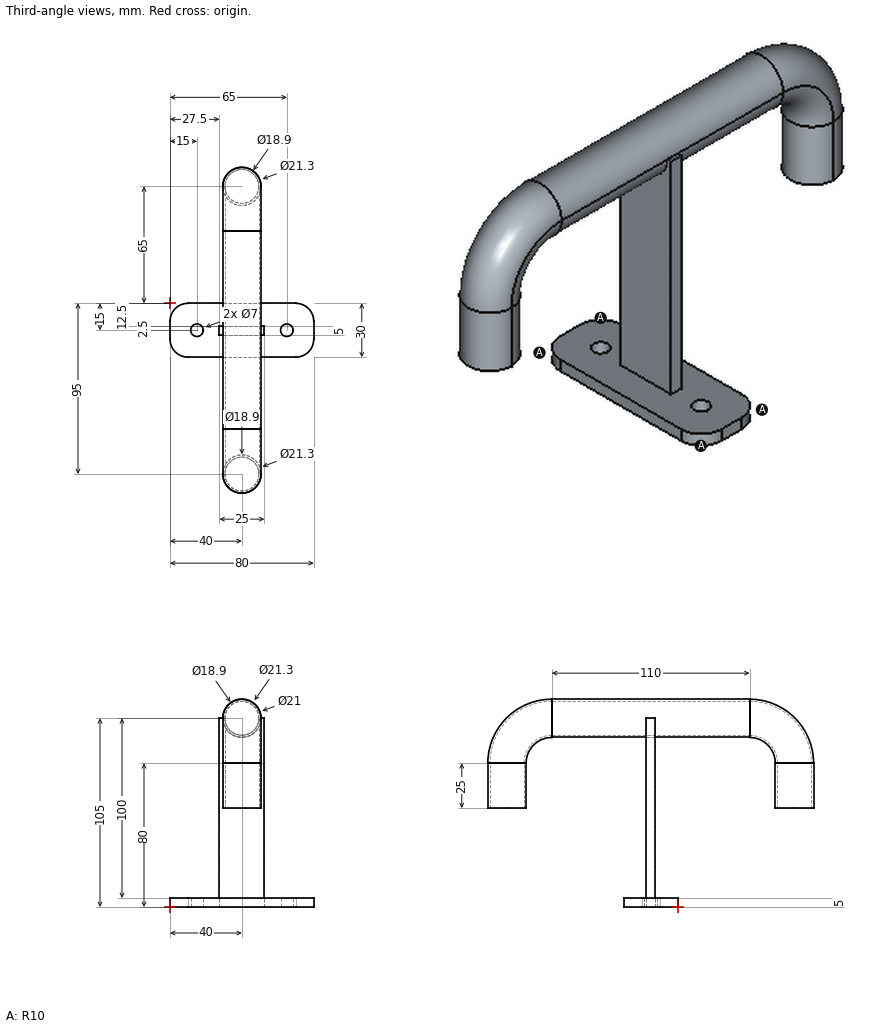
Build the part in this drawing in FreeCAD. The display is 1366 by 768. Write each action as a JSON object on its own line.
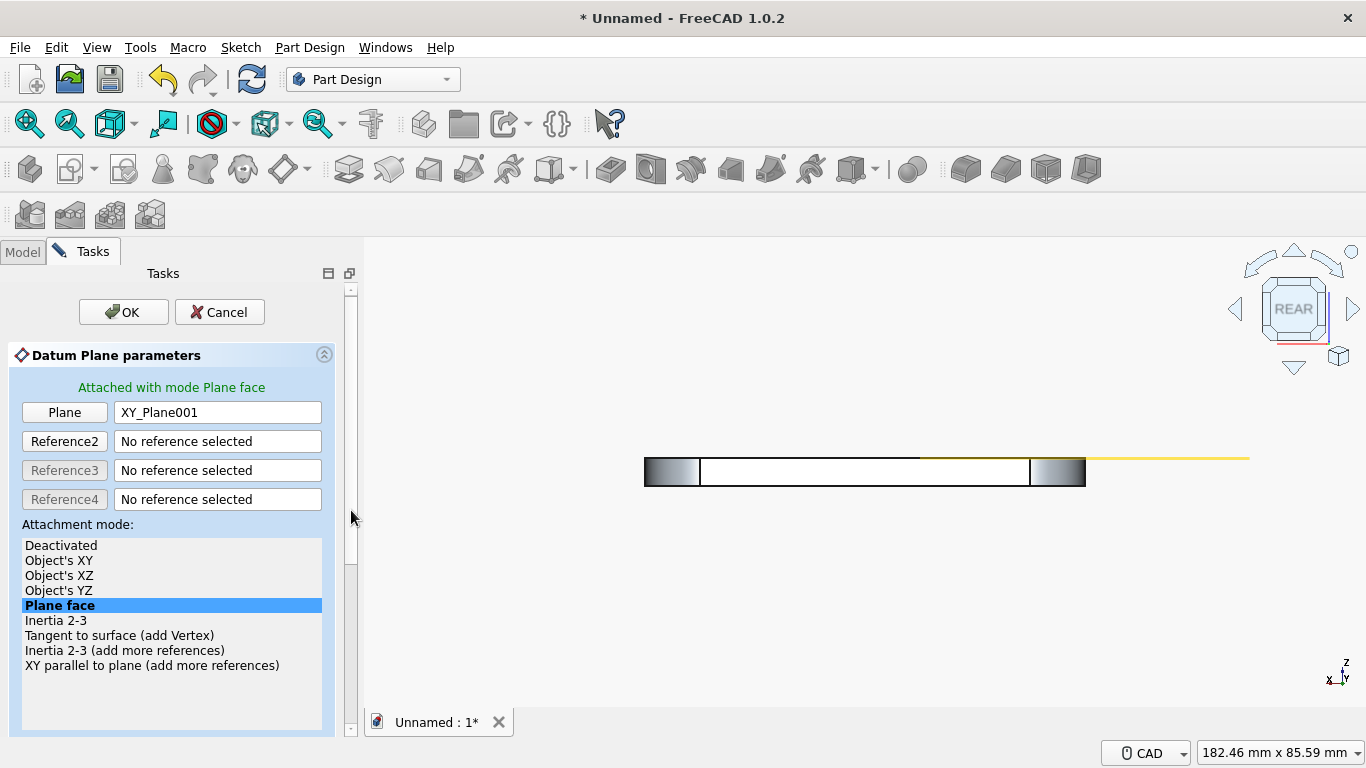
{"action": "left_click", "coordinate": [124, 312]}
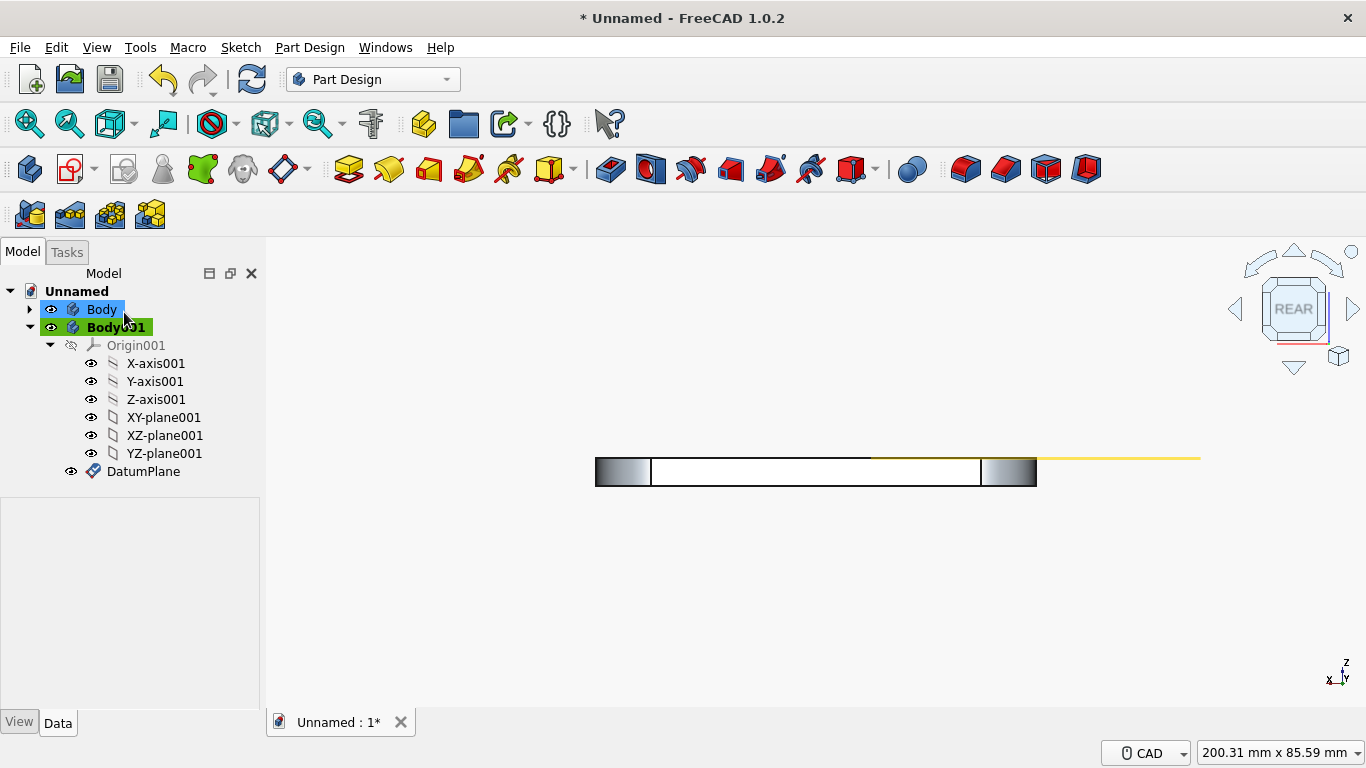
{"action": "left_click", "coordinate": [116, 471]}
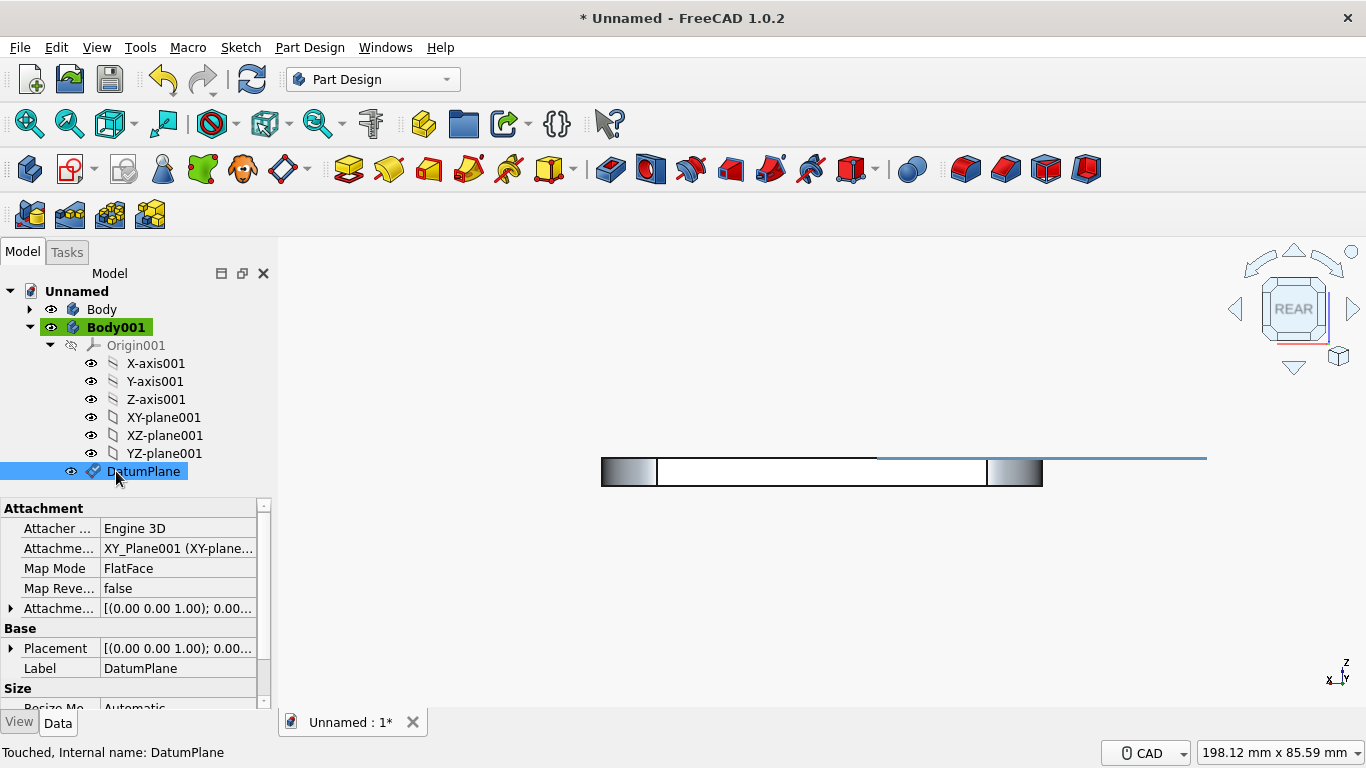
{"action": "left_click", "coordinate": [70, 170]}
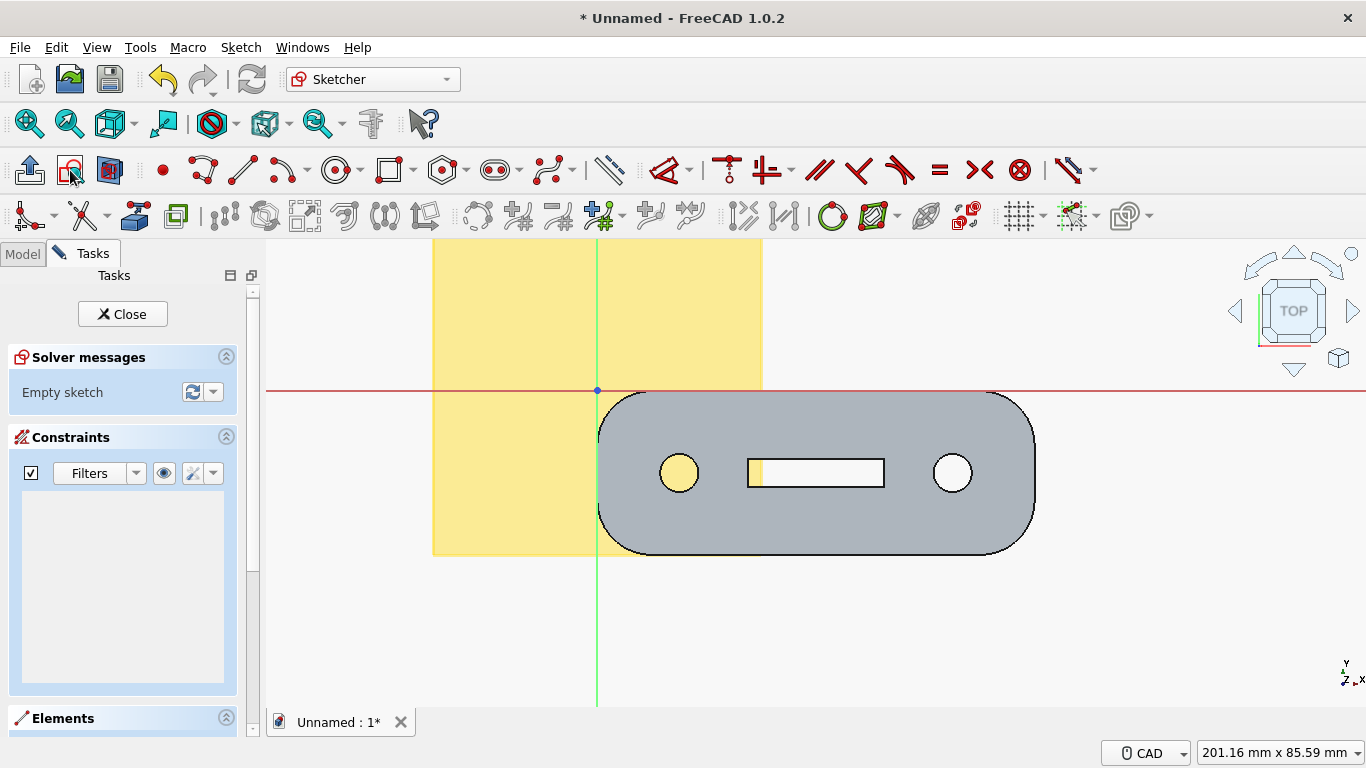
{"action": "scroll", "coordinate": [735, 411], "scroll_direction": "up", "scroll_amount": 4}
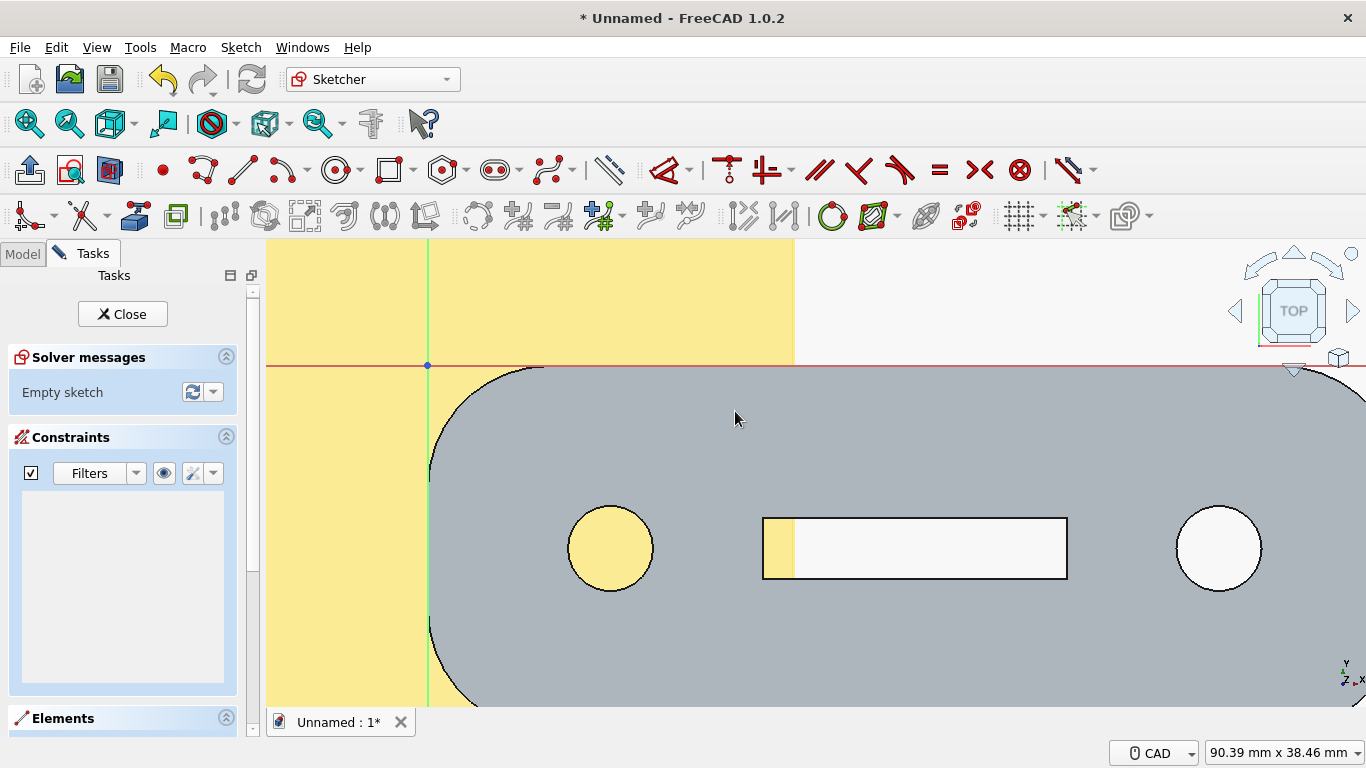
{"action": "left_click", "coordinate": [390, 170]}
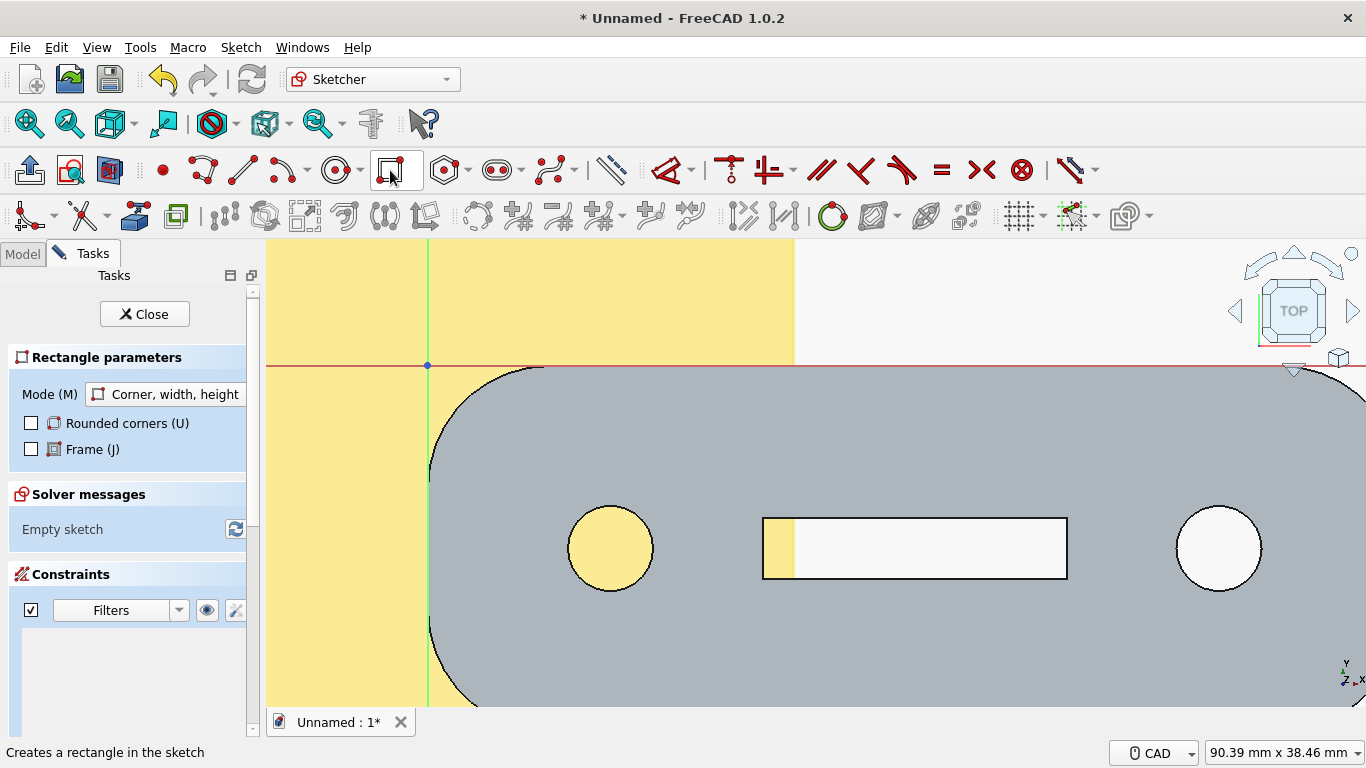
{"action": "left_click", "coordinate": [763, 518]}
{"action": "mouse_move", "coordinate": [1067, 579]}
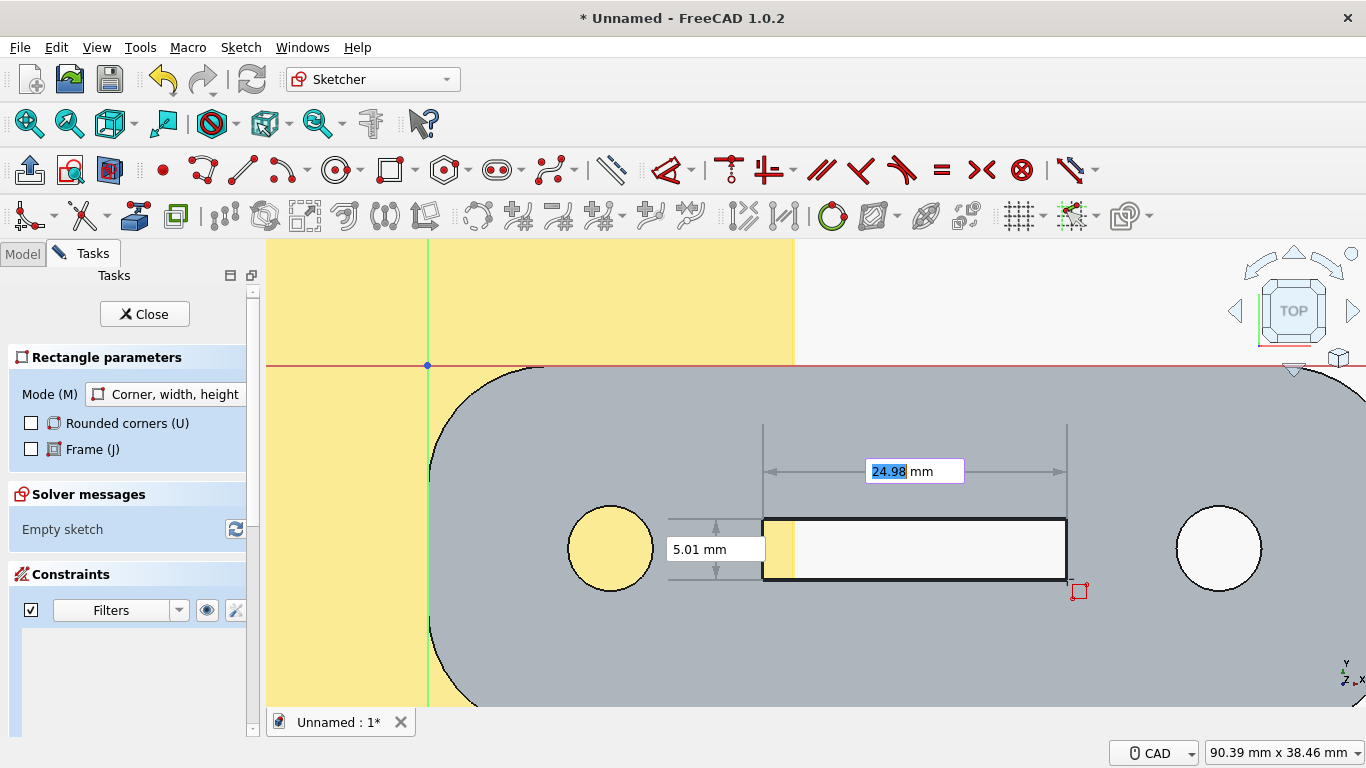
{"action": "type", "text": "25"}
{"action": "key", "text": "Tab"}
{"action": "type", "text": "5"}
{"action": "key", "text": "Return"}
{"action": "key", "text": "Escape"}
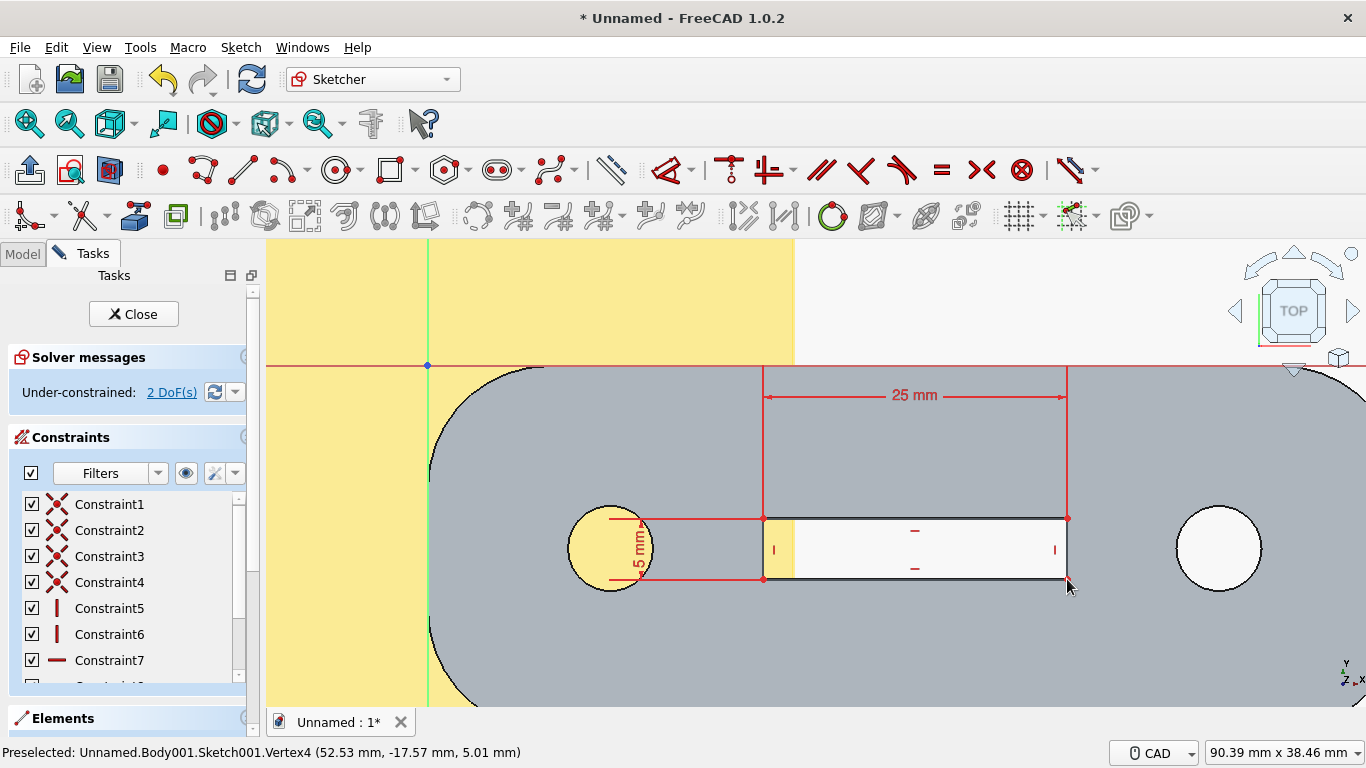
{"action": "left_click", "coordinate": [666, 170]}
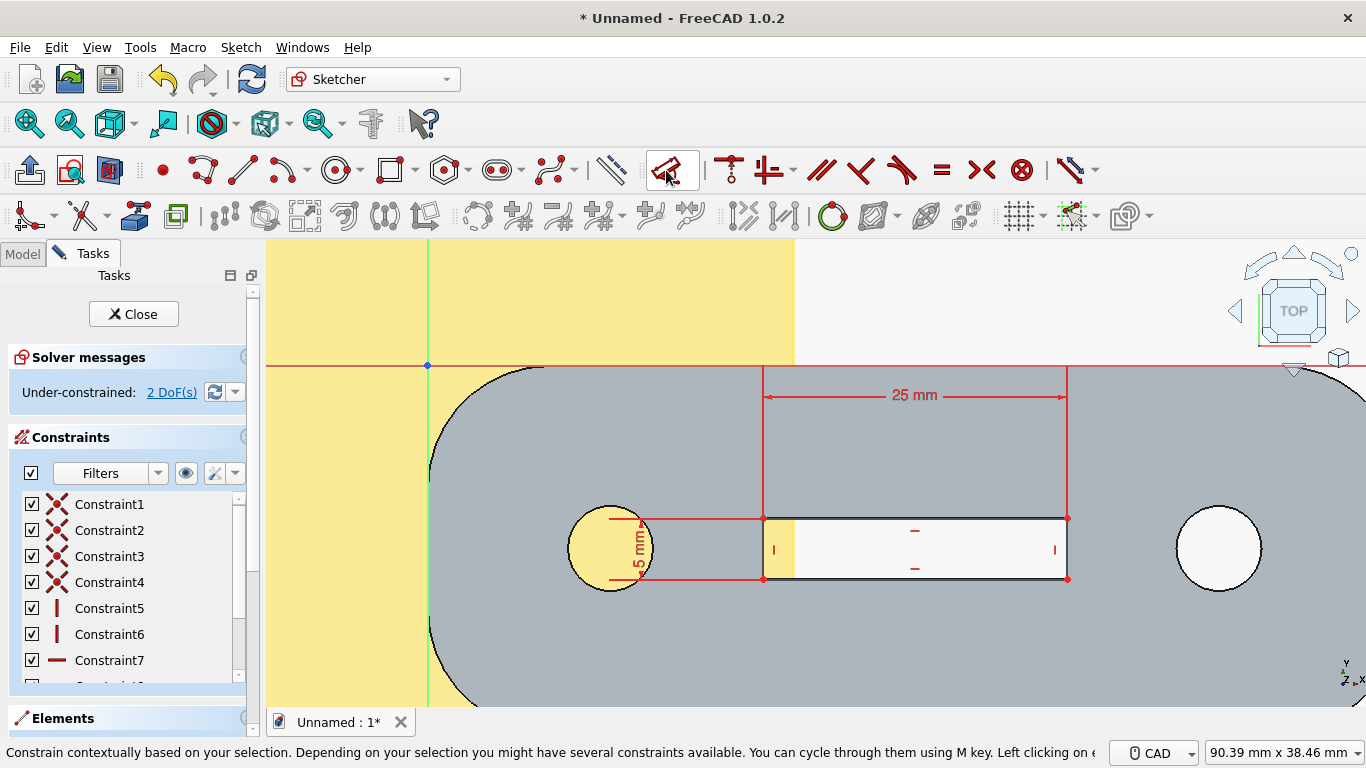
{"action": "left_click", "coordinate": [763, 519]}
{"action": "left_click", "coordinate": [595, 332]}